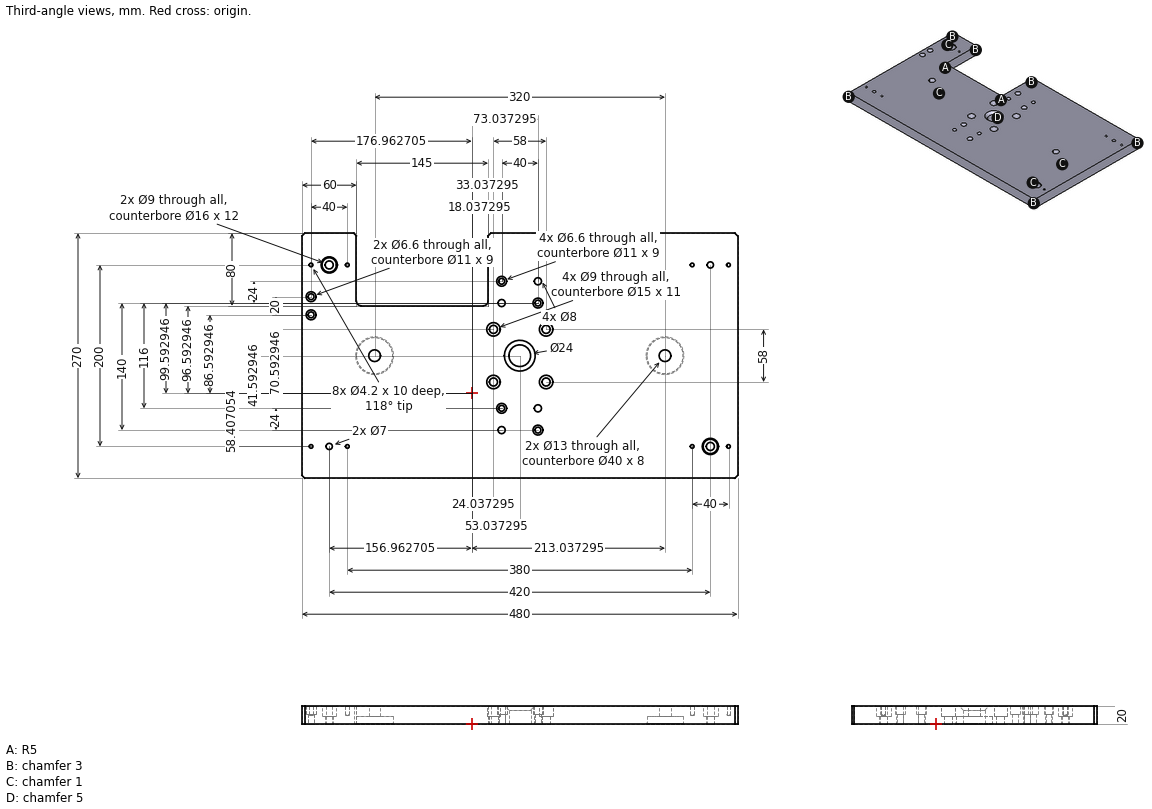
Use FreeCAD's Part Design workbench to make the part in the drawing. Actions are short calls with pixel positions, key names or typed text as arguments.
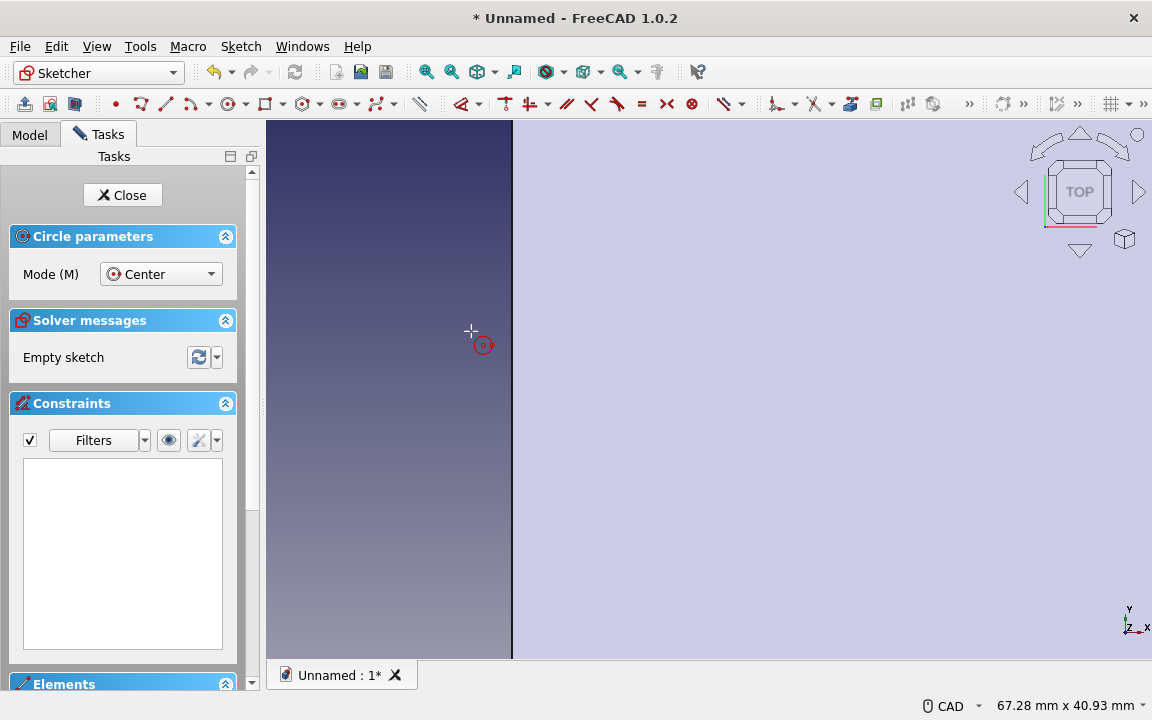
click(644, 258)
click(674, 227)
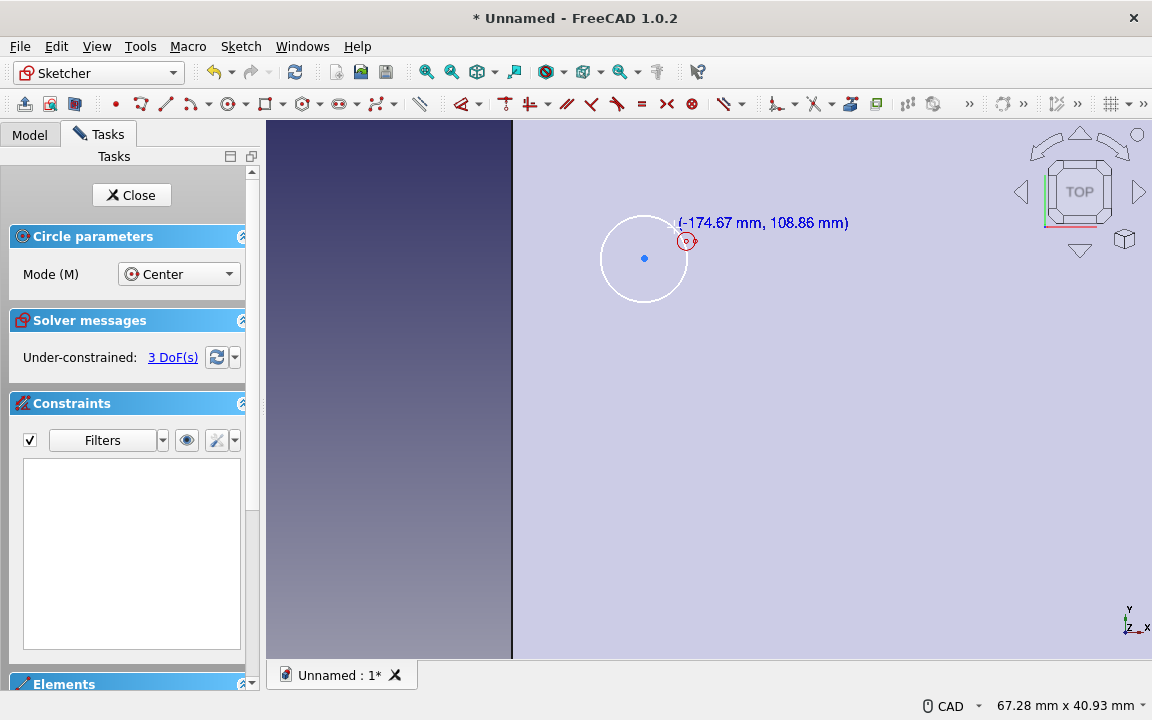
click(644, 521)
click(674, 490)
key(Escape)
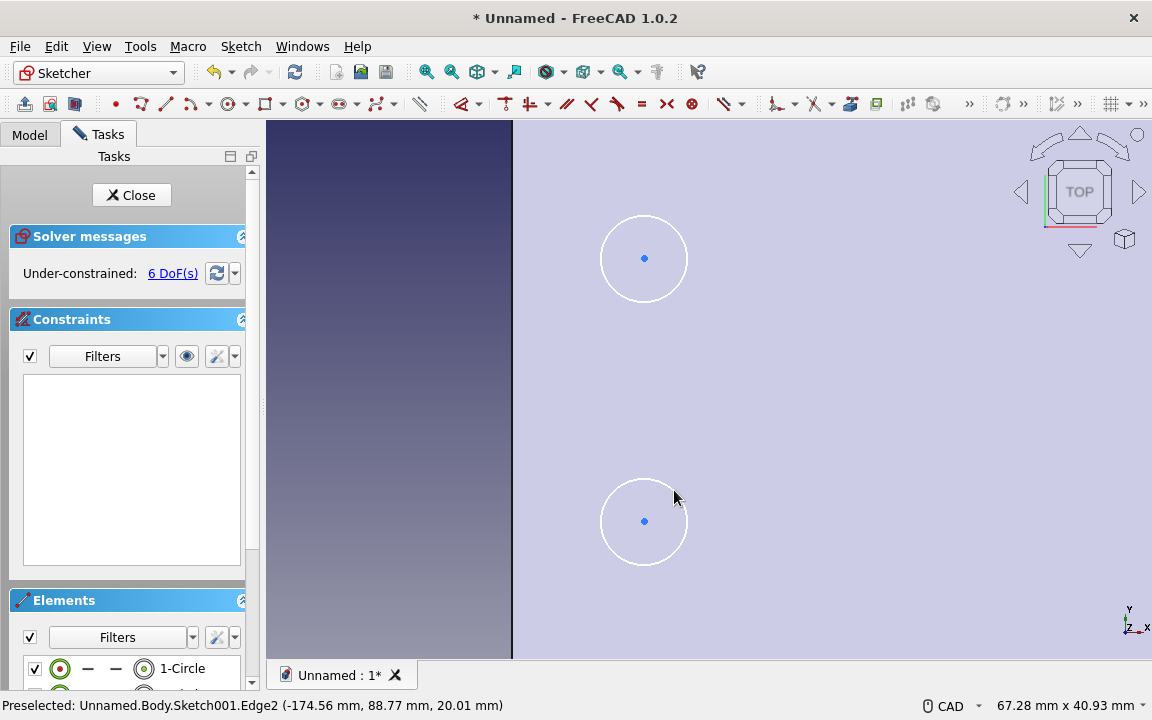
click(674, 228)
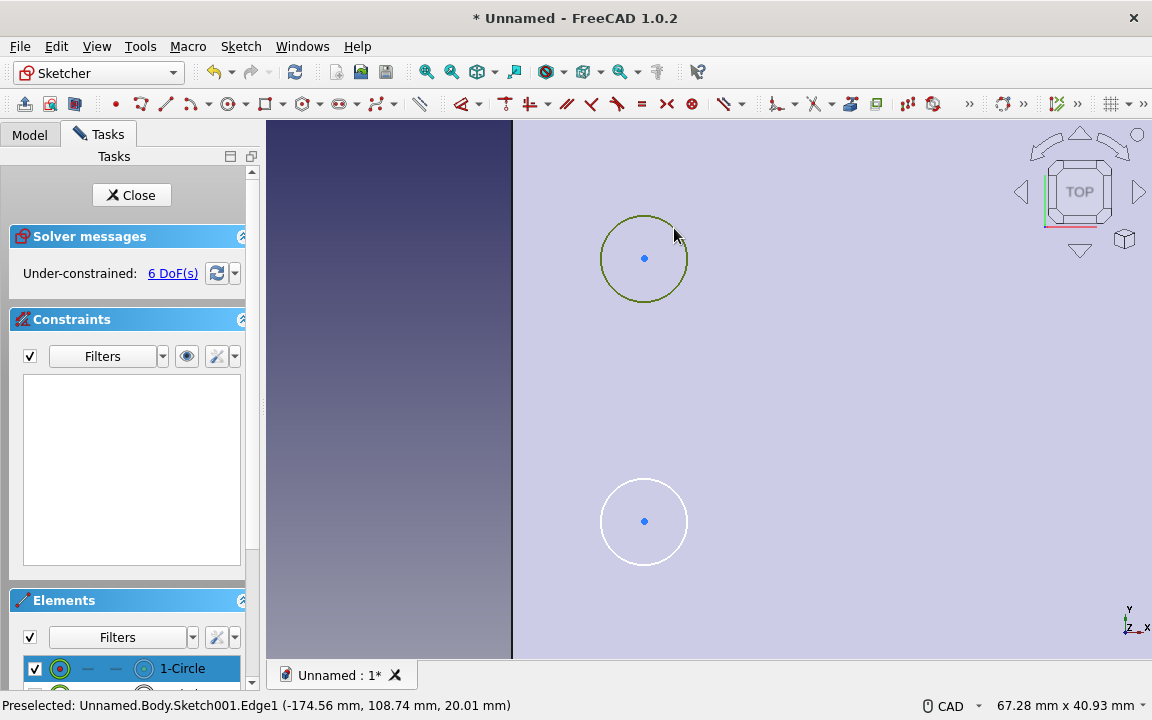
click(674, 491)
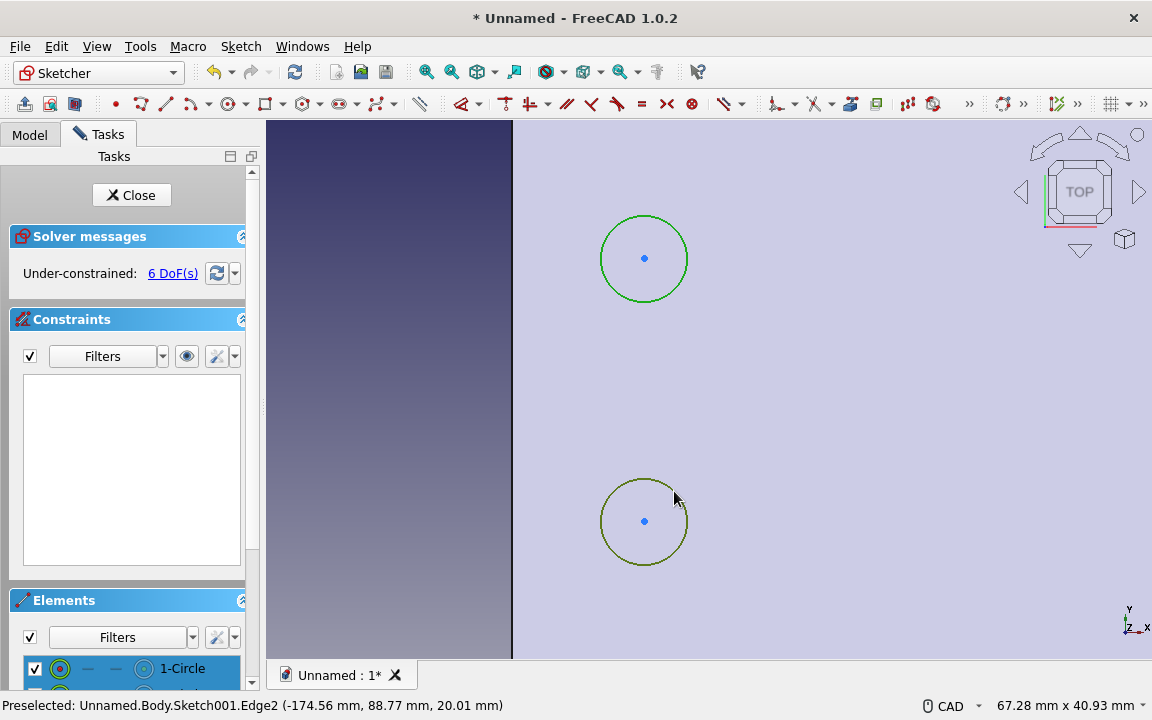
key(e)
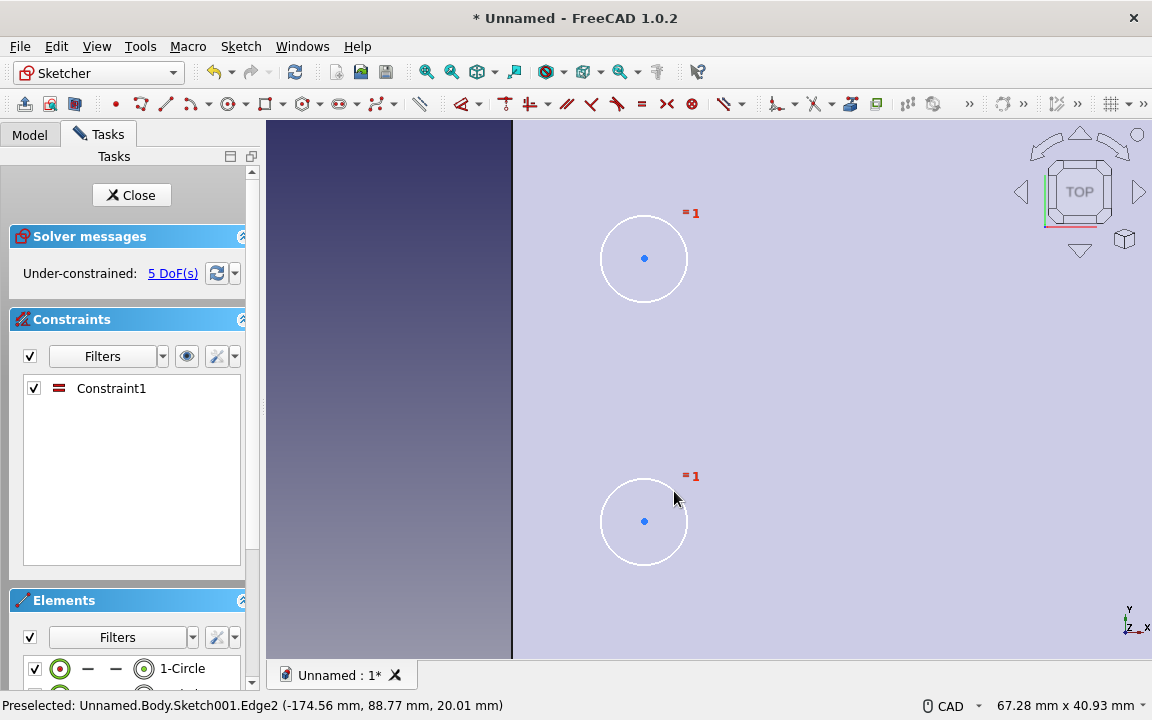
click(644, 259)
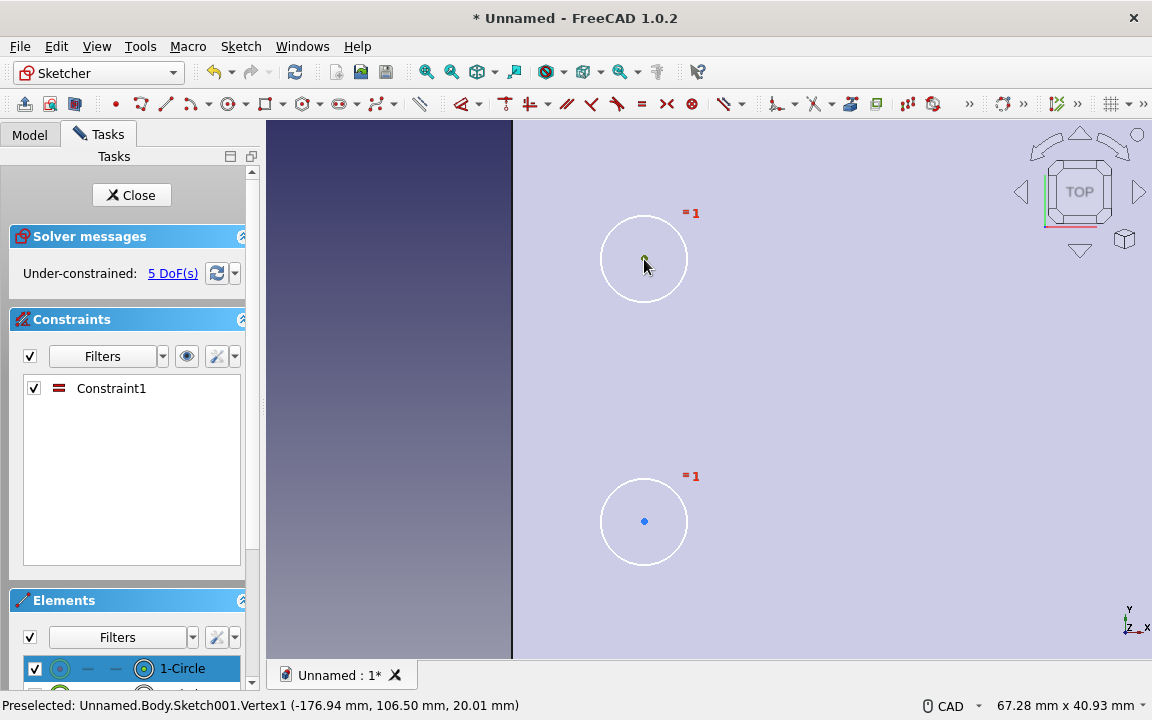
click(644, 522)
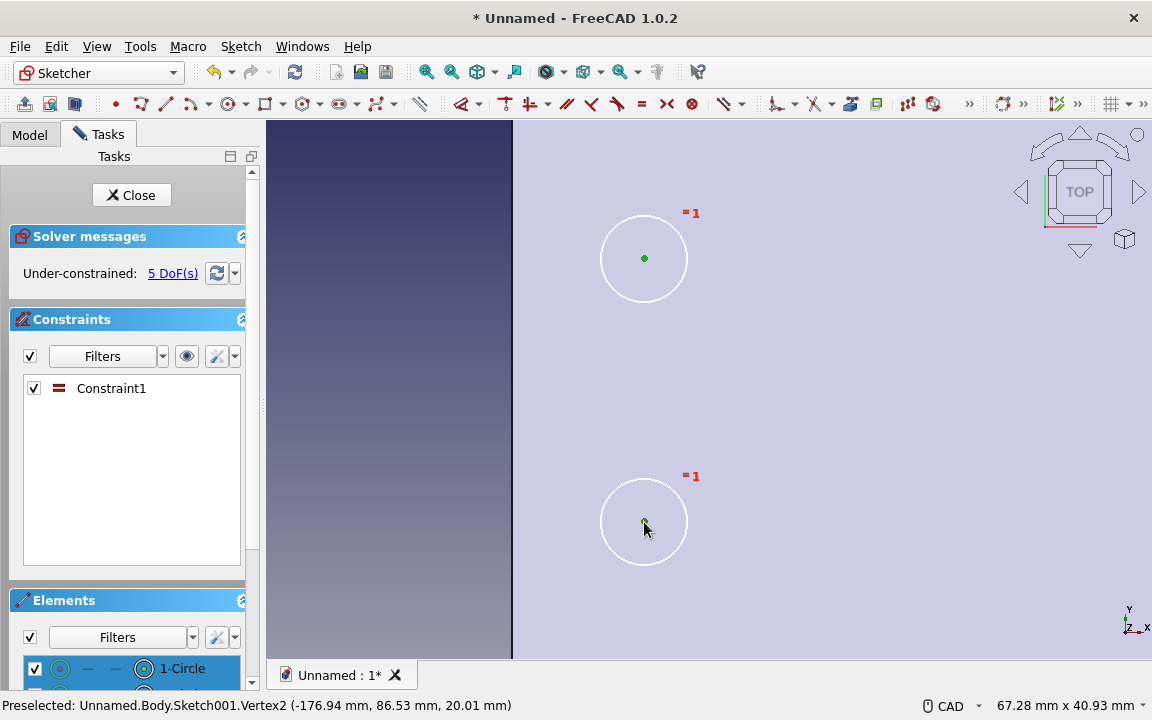
click(548, 104)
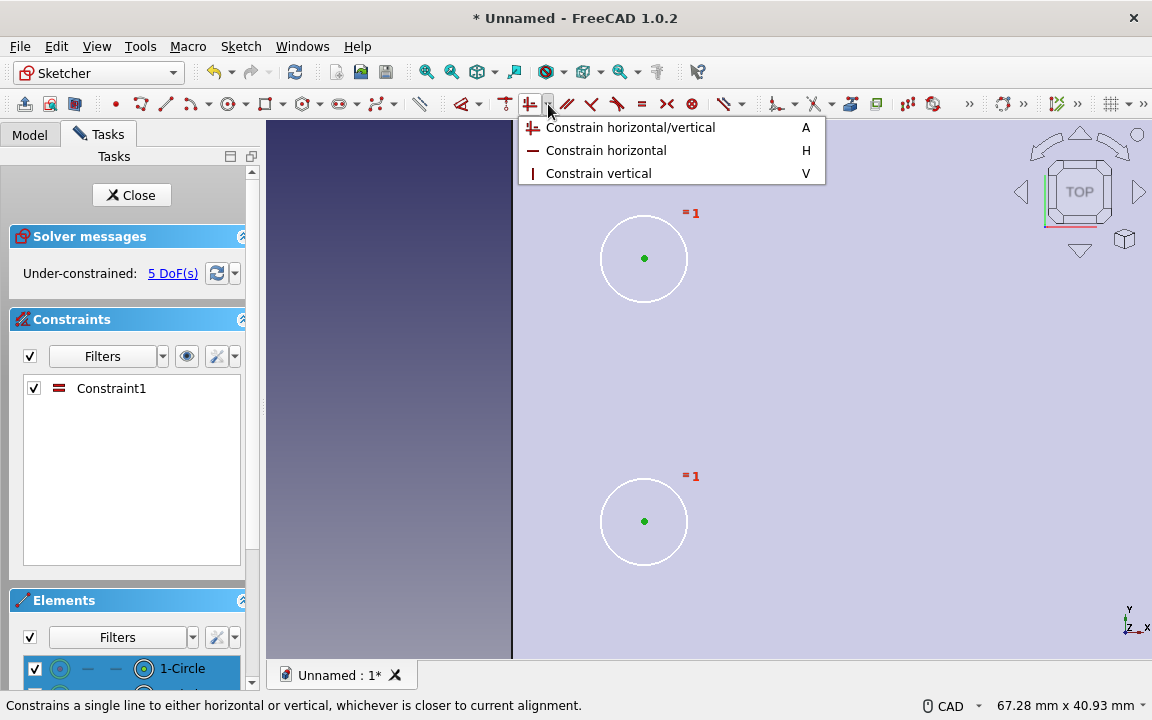
click(672, 174)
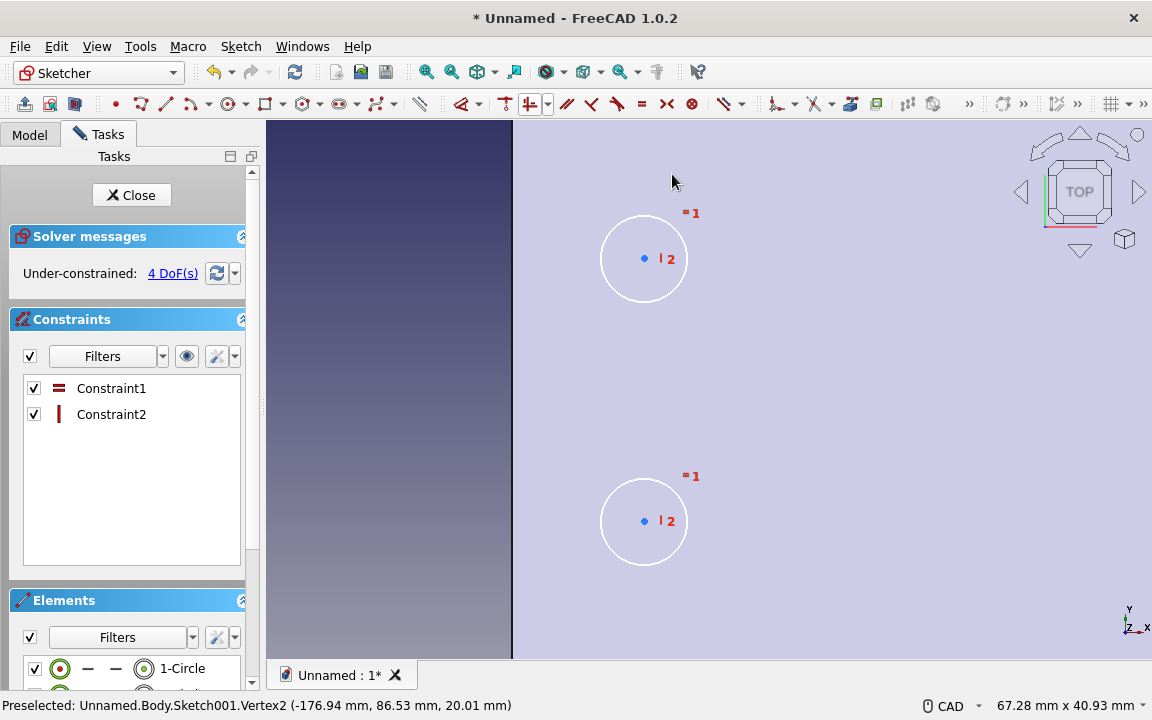
click(460, 104)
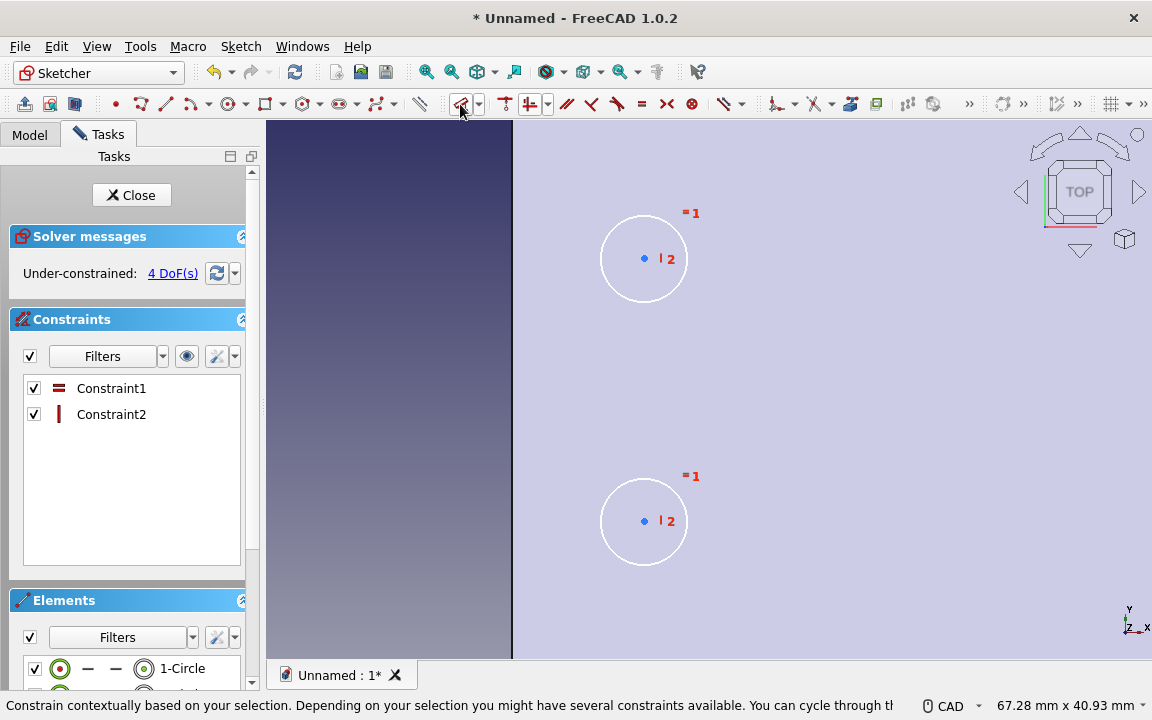
click(674, 228)
click(696, 205)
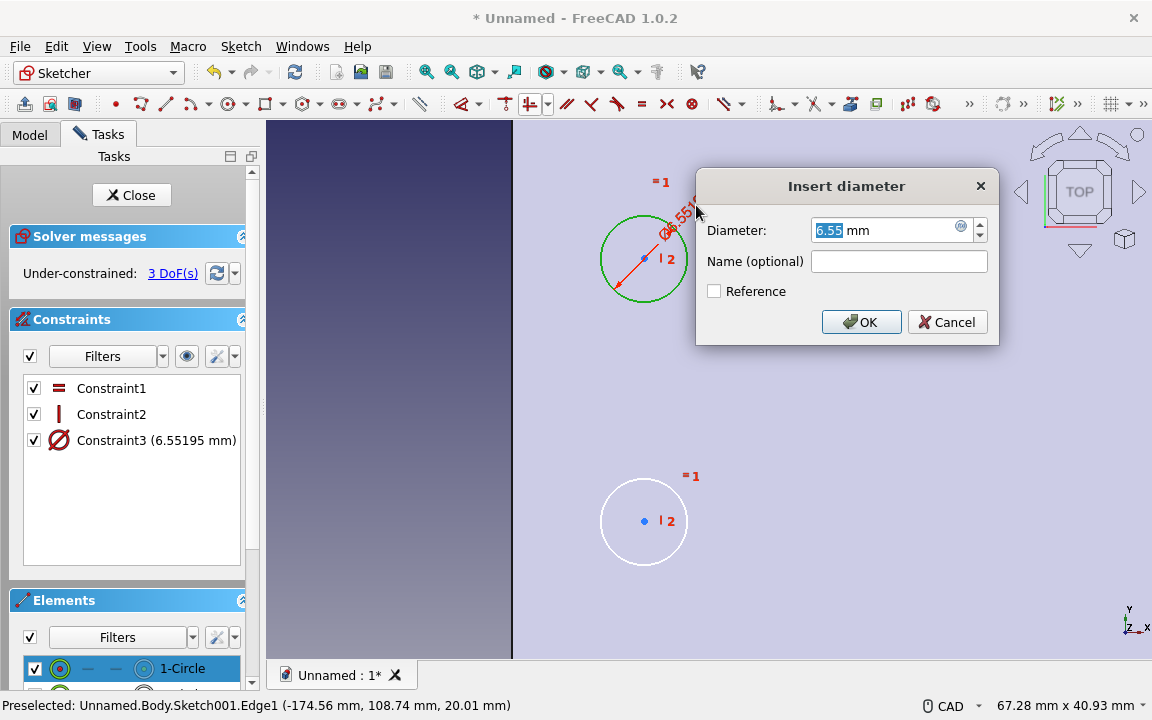
text(6.6)
key(Return)